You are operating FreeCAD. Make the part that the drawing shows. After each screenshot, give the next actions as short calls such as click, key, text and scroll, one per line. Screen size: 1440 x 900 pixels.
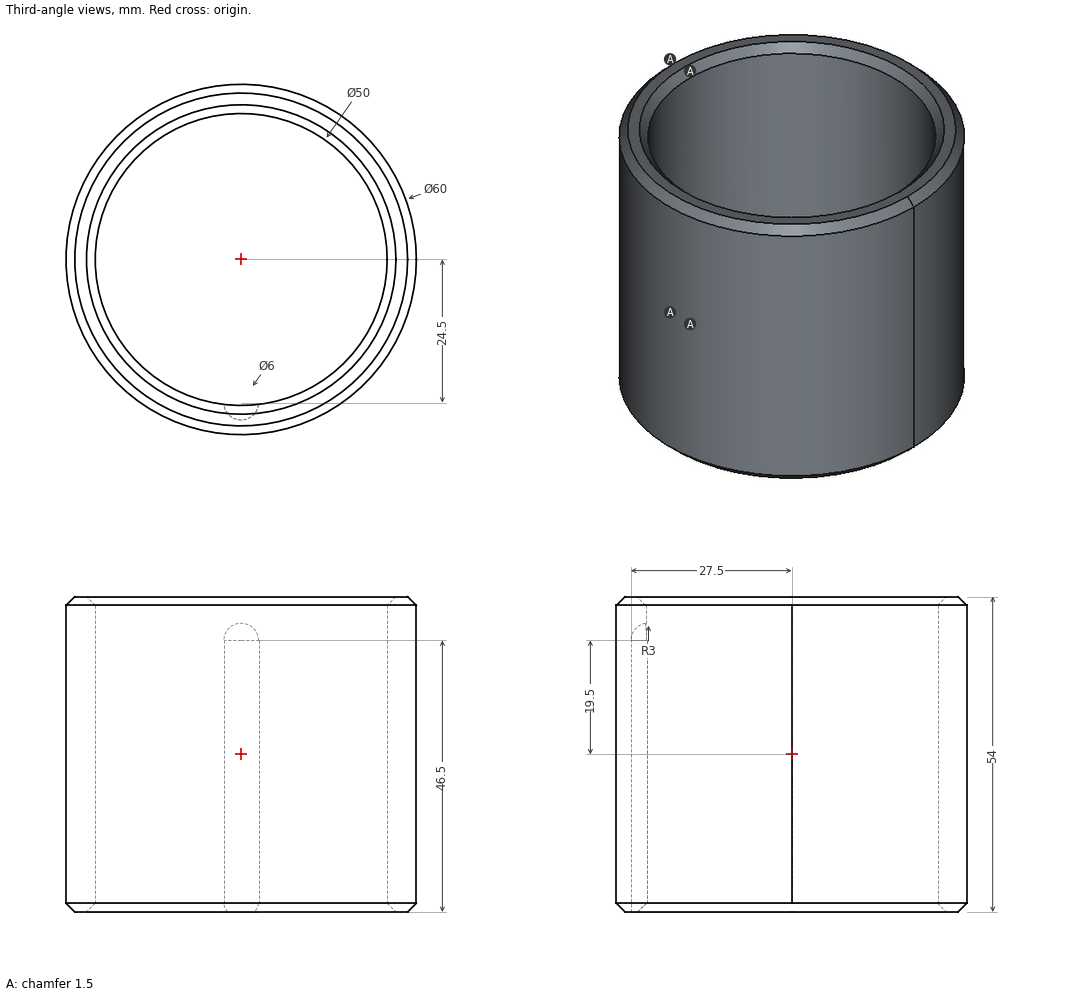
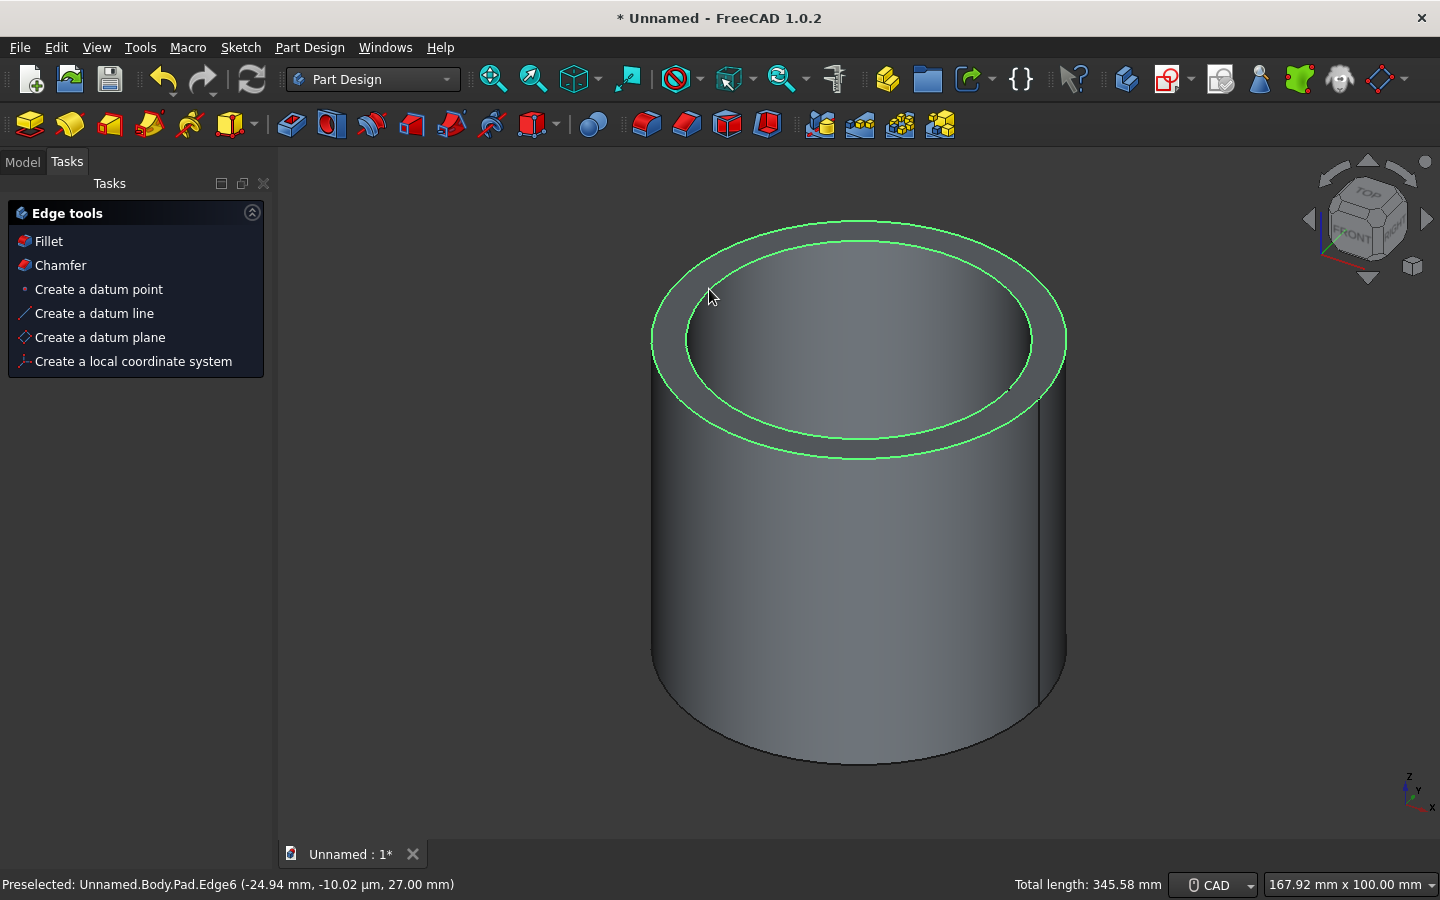
key(0)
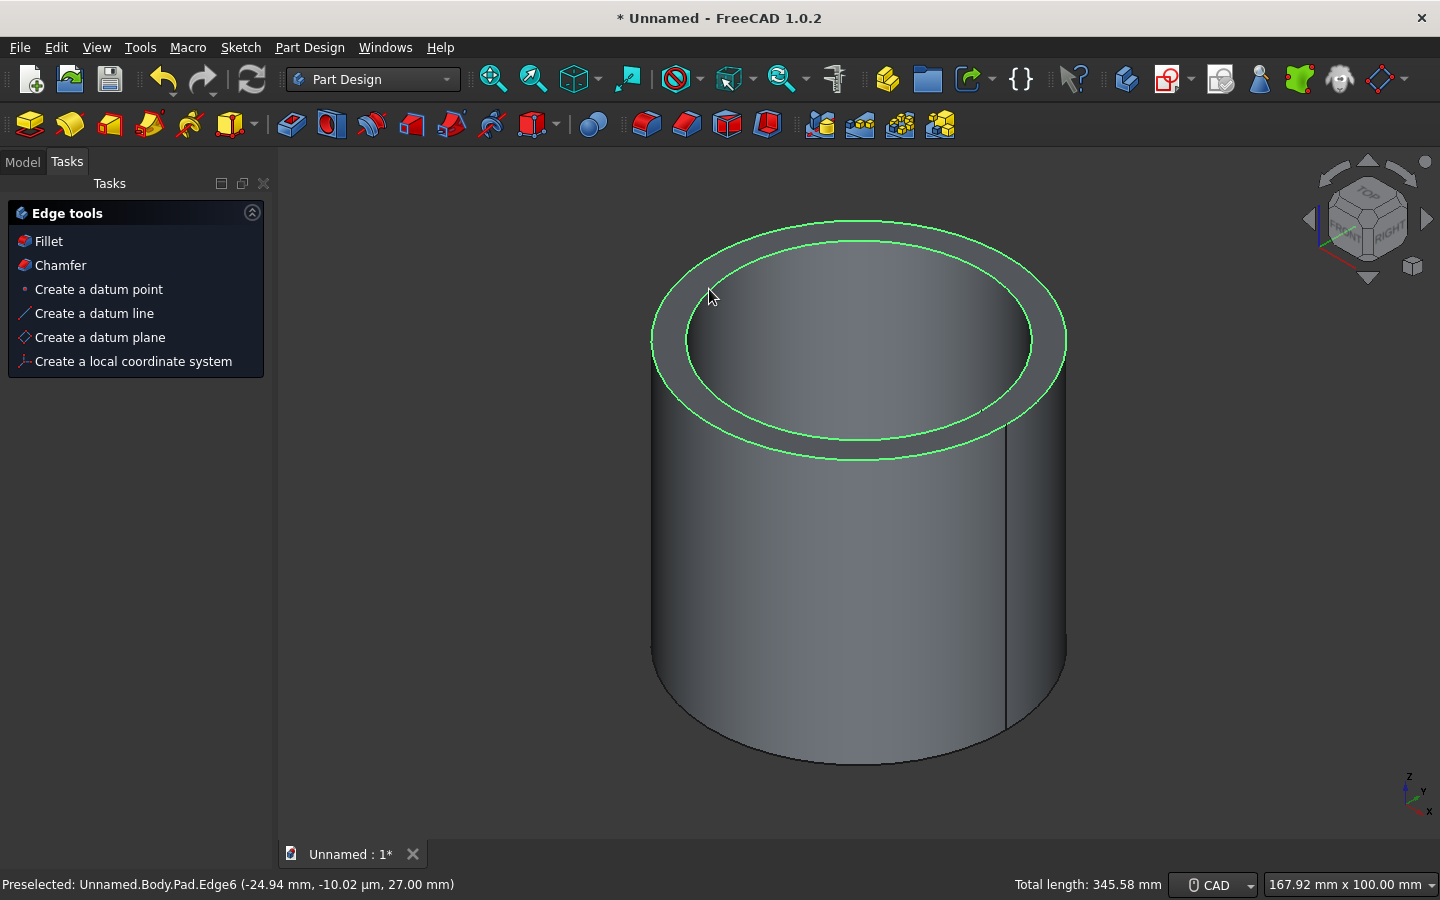
key(2)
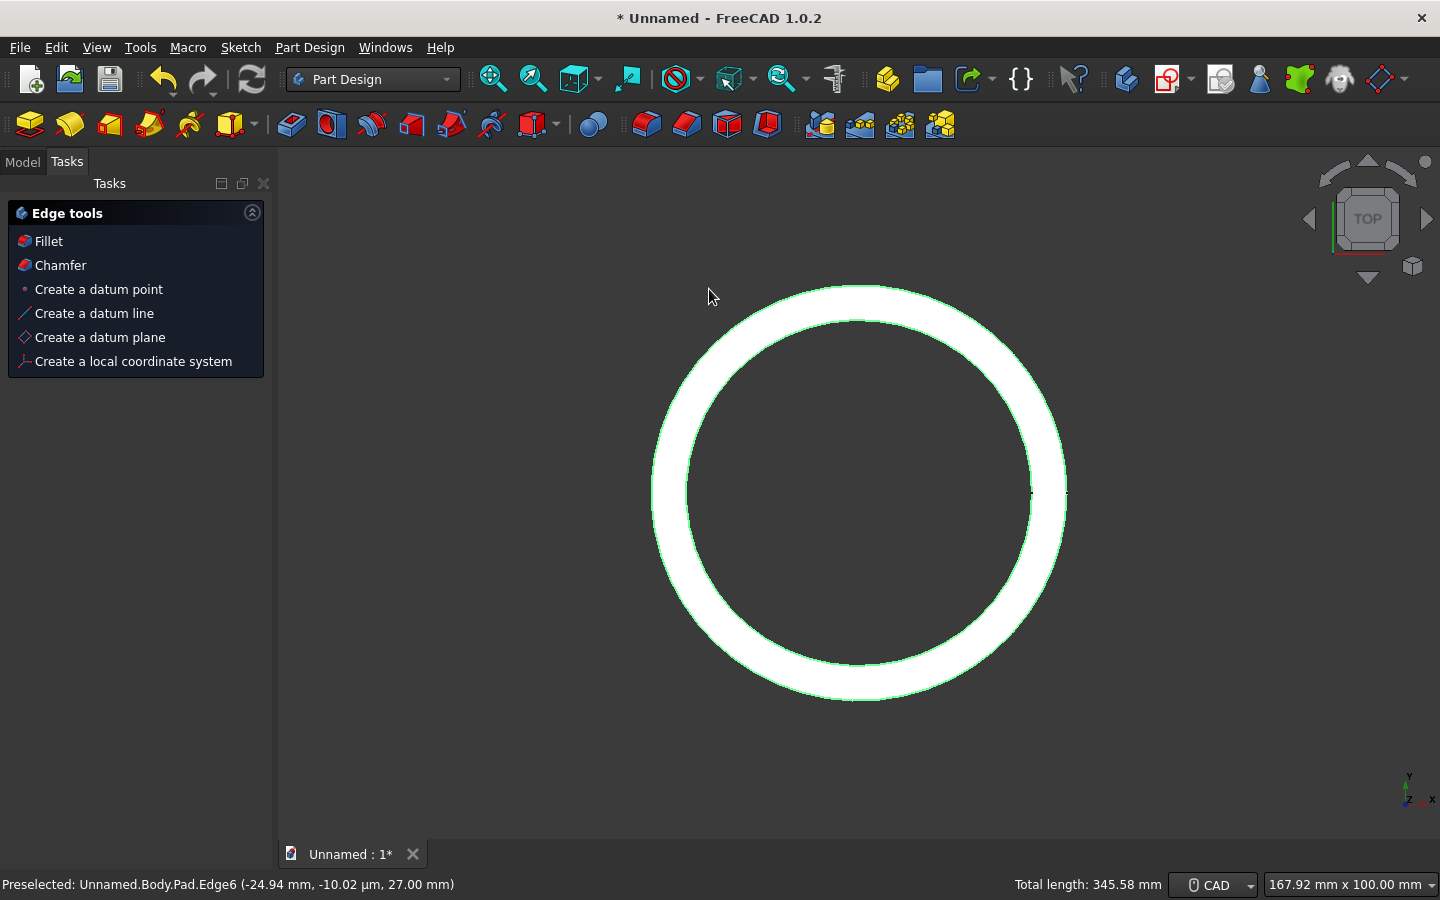
key(1)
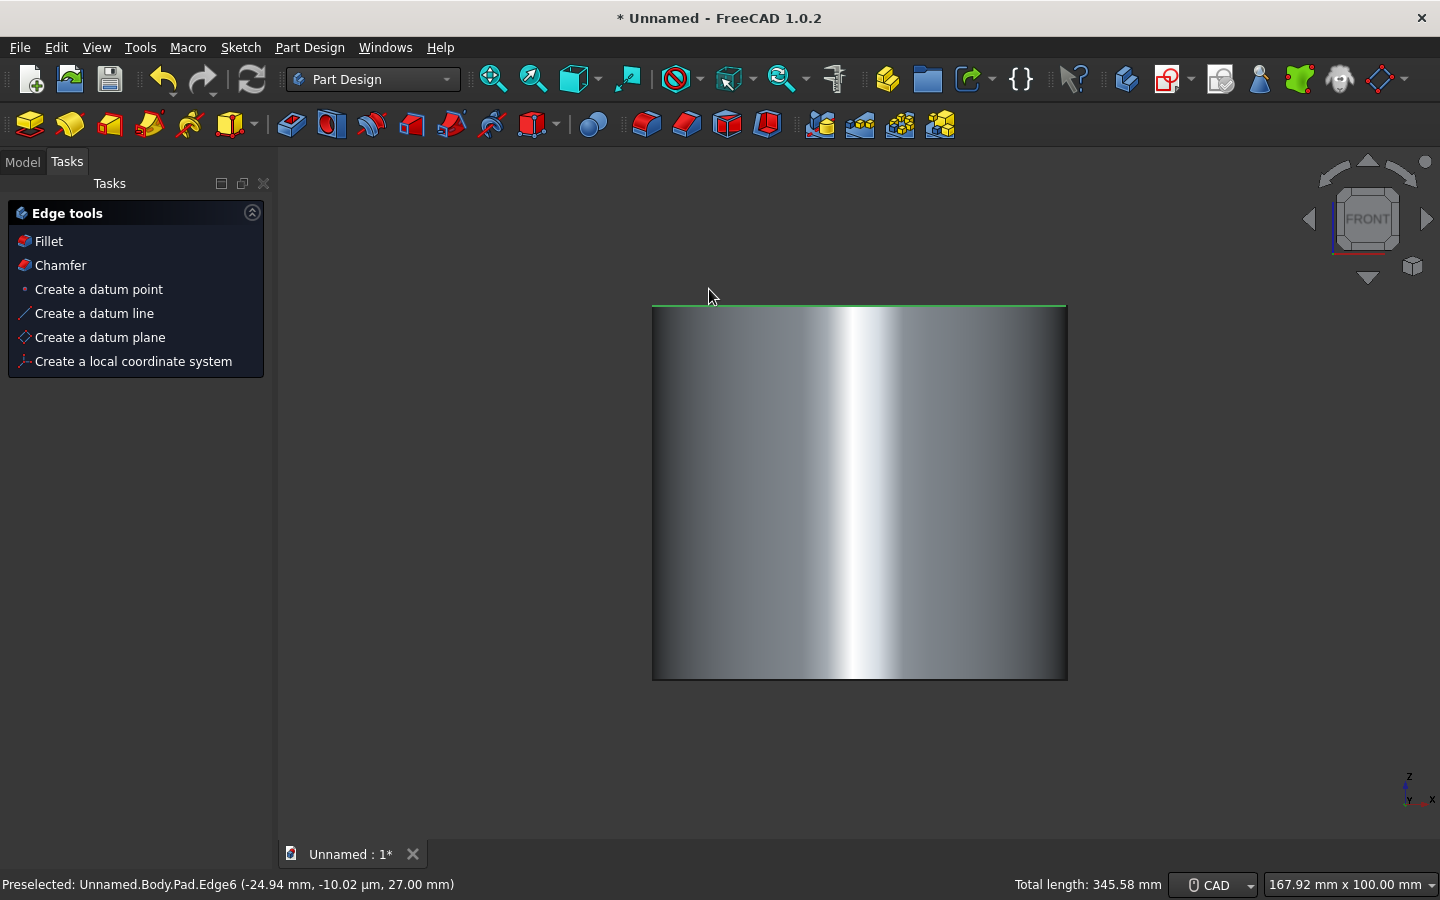
click(691, 679, ctrl)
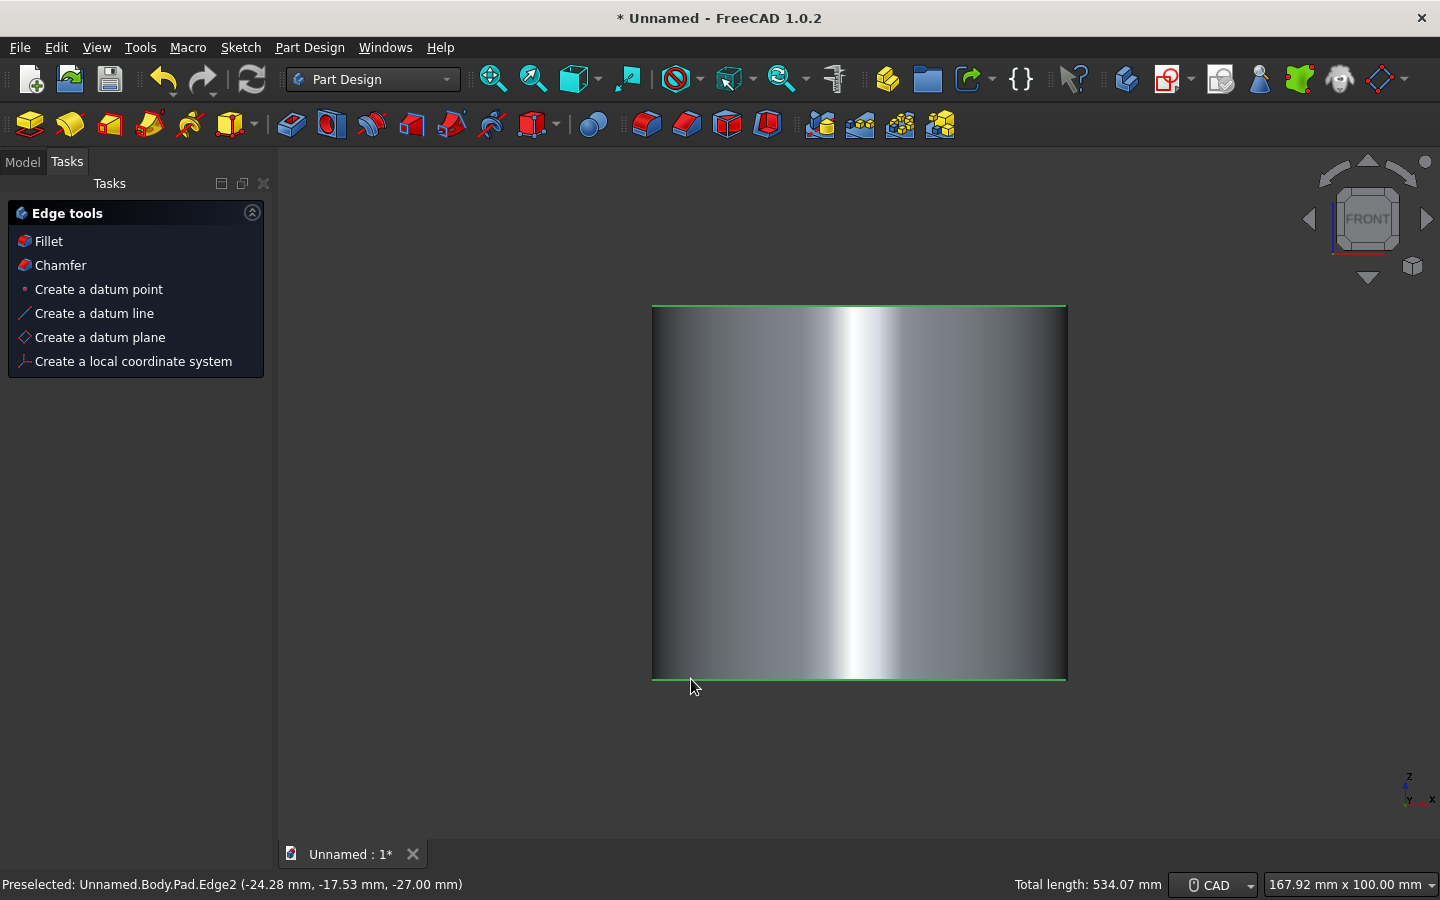
key(3)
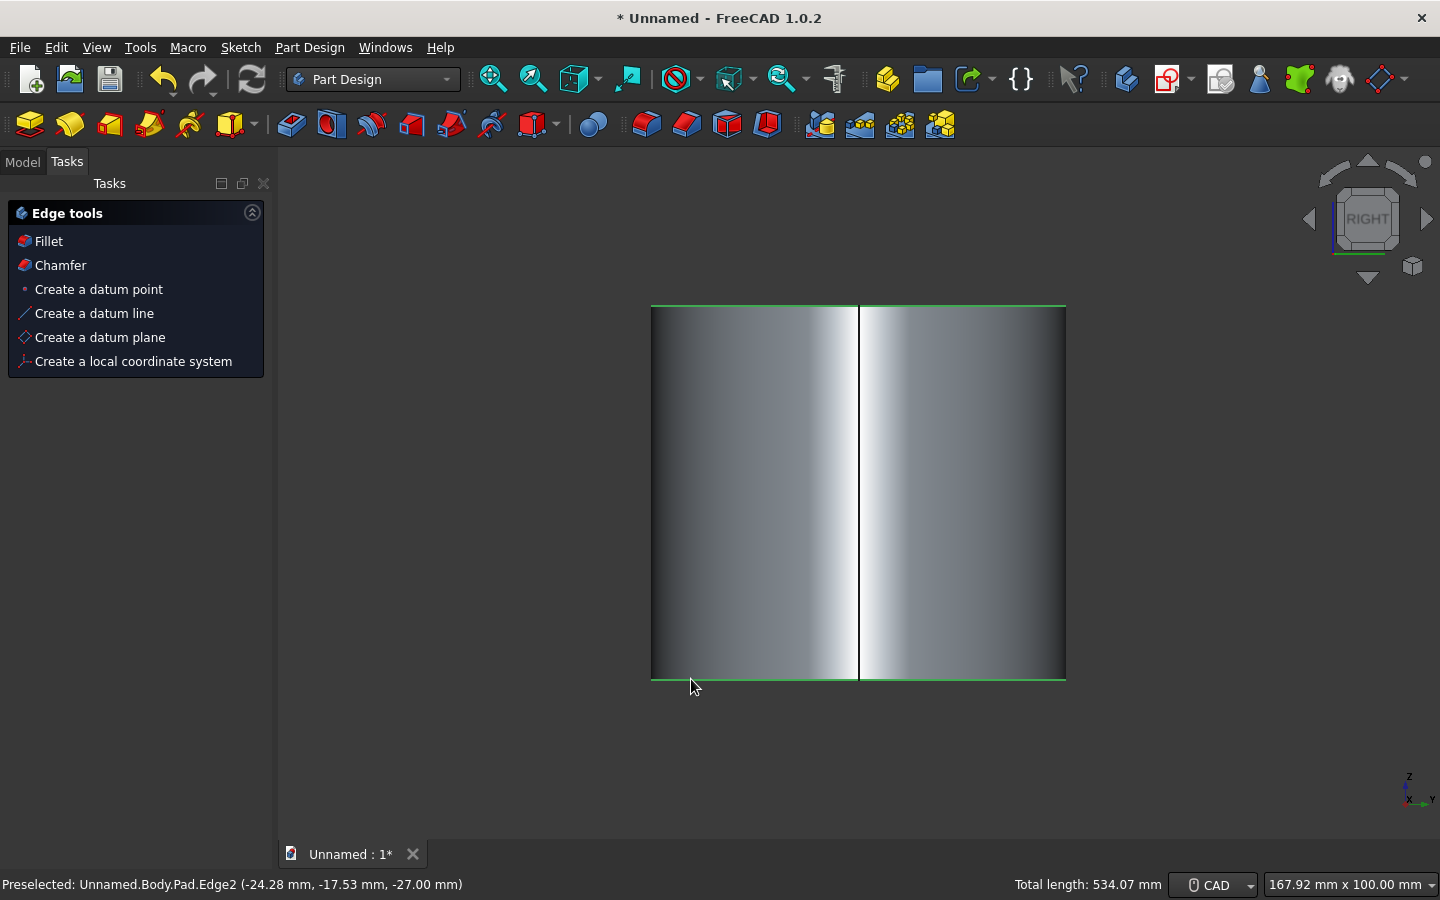
key(5)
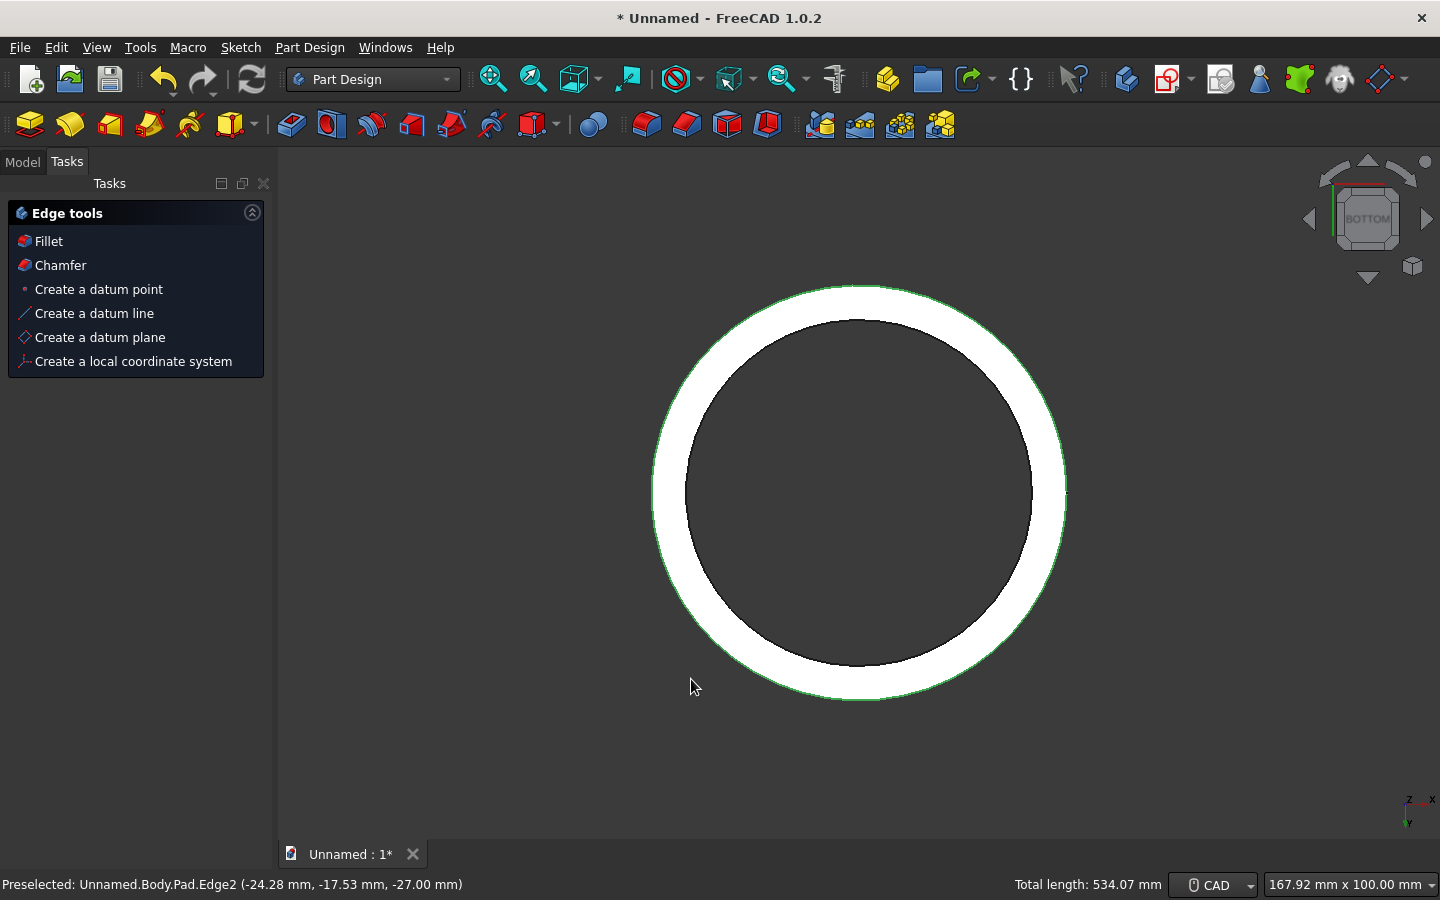
click(686, 492, ctrl)